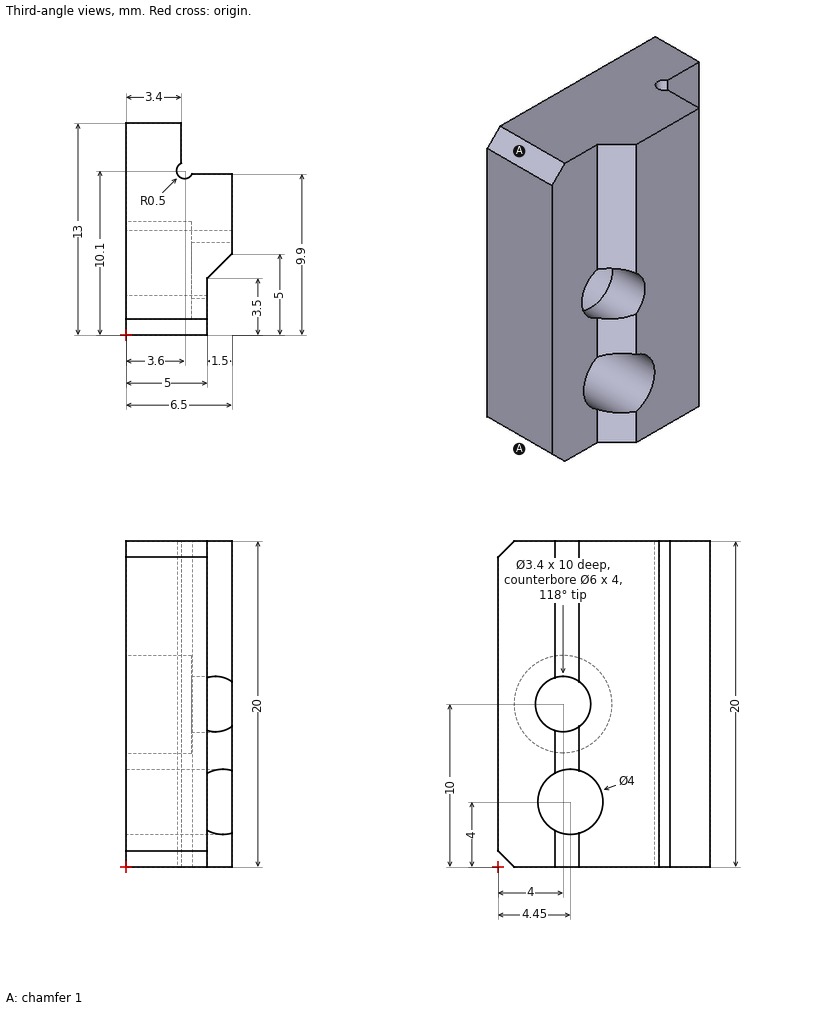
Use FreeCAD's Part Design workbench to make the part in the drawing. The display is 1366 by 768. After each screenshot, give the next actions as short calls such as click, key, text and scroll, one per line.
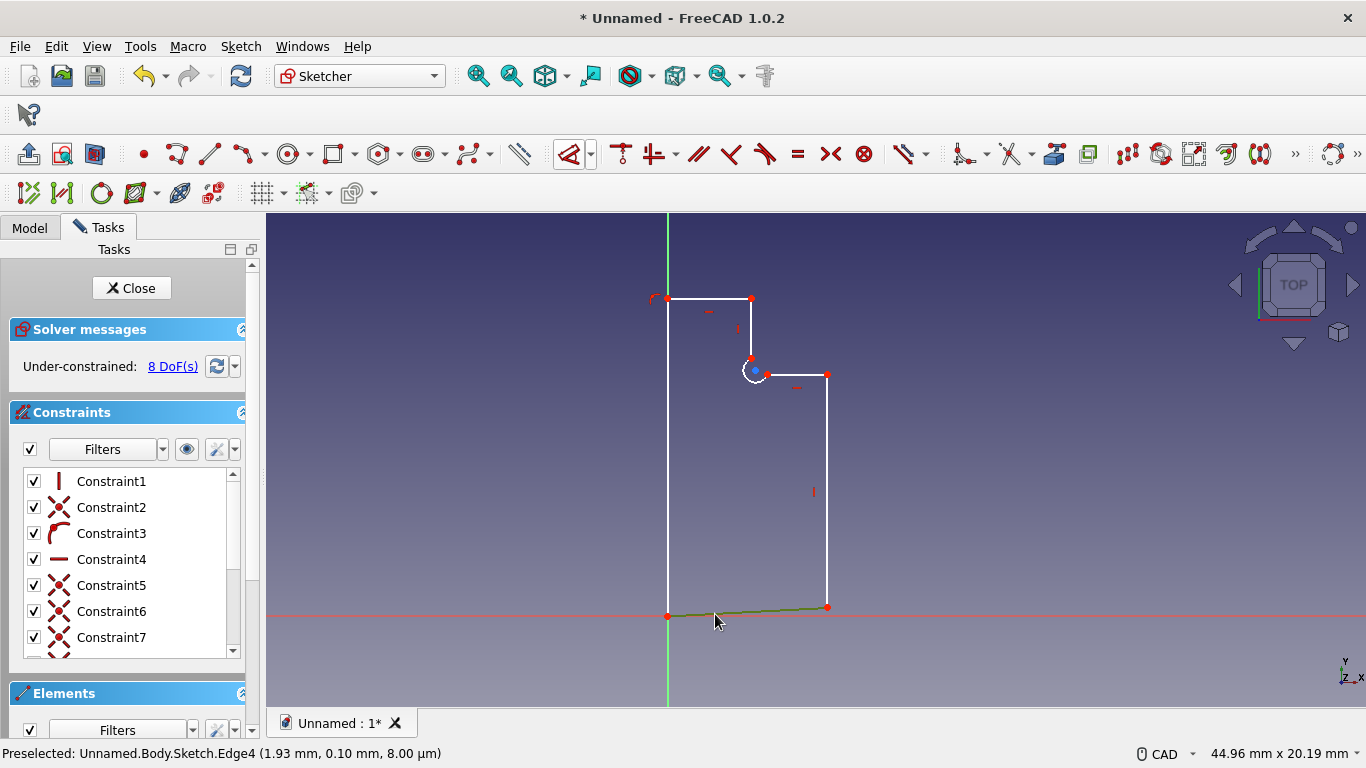
key(h)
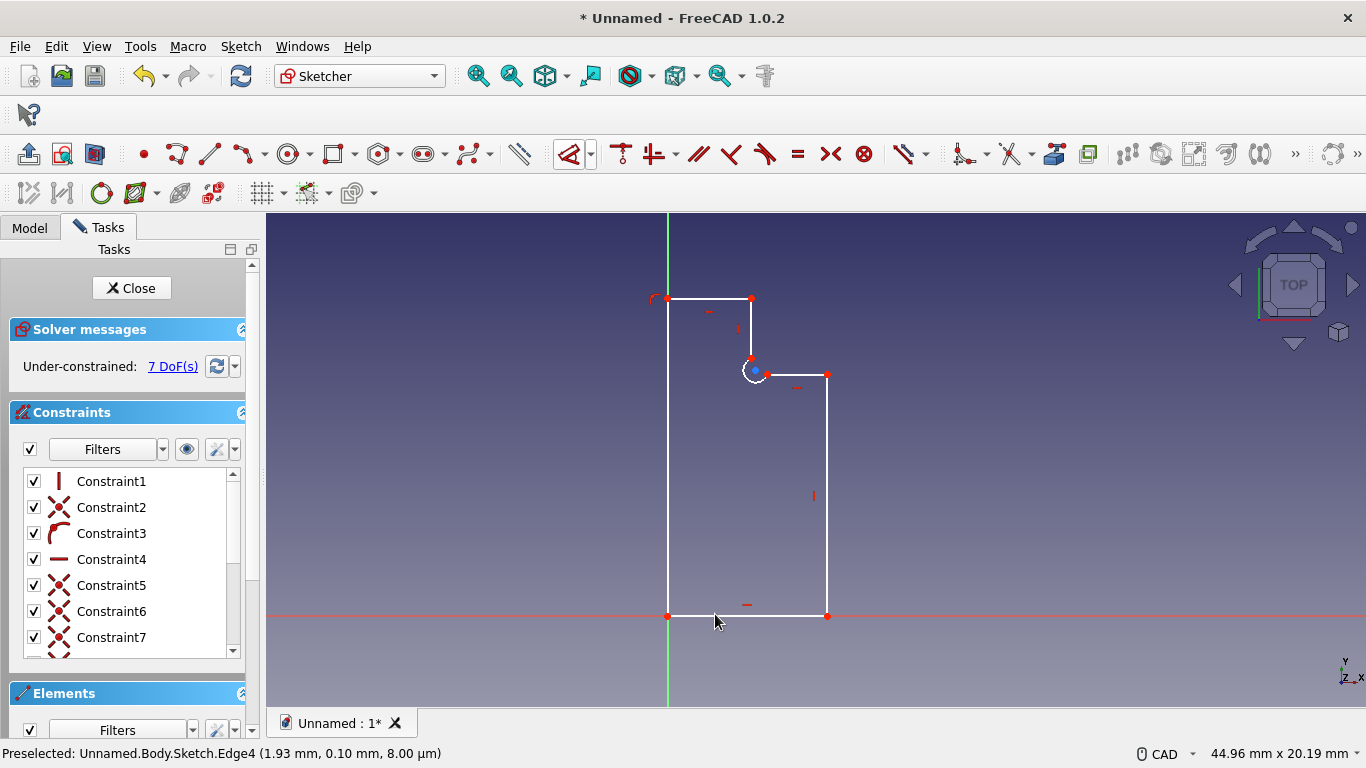
click(568, 154)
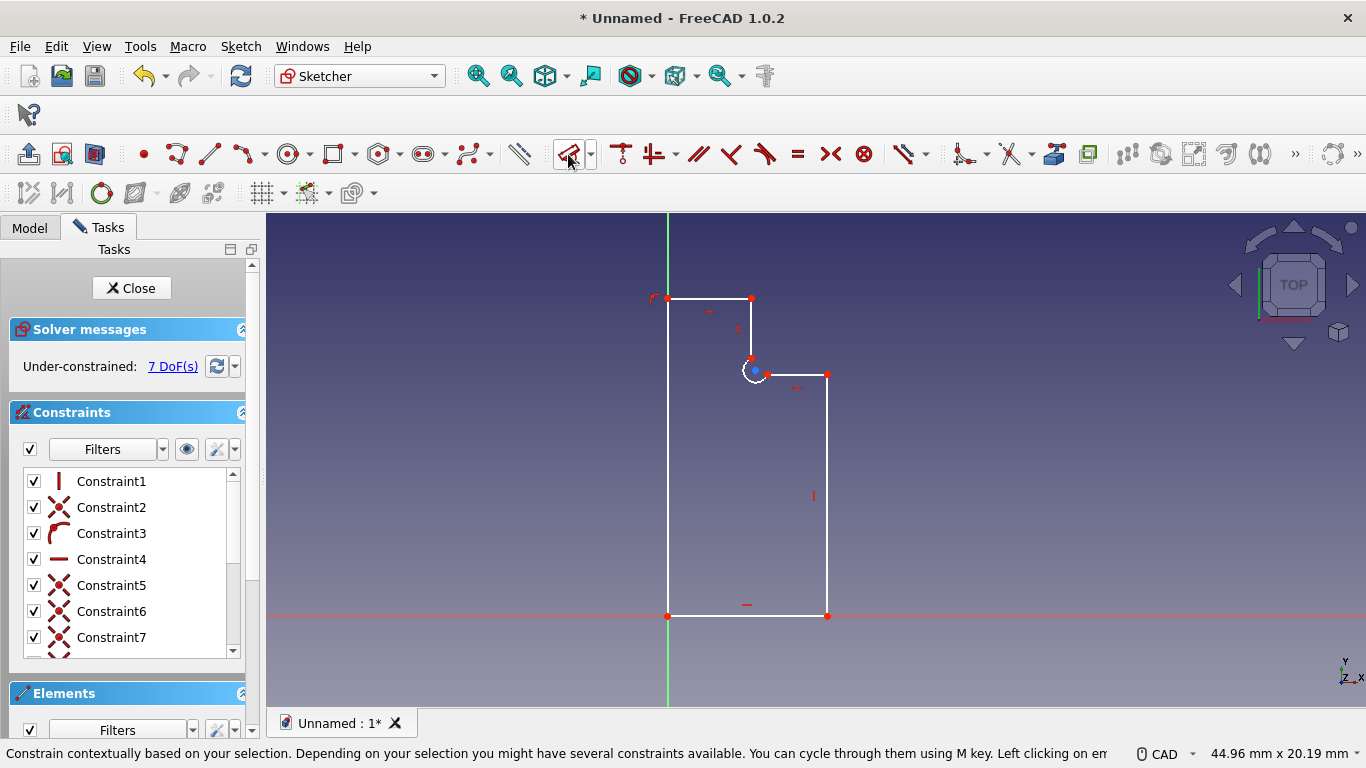
scroll(743, 370, up, 6)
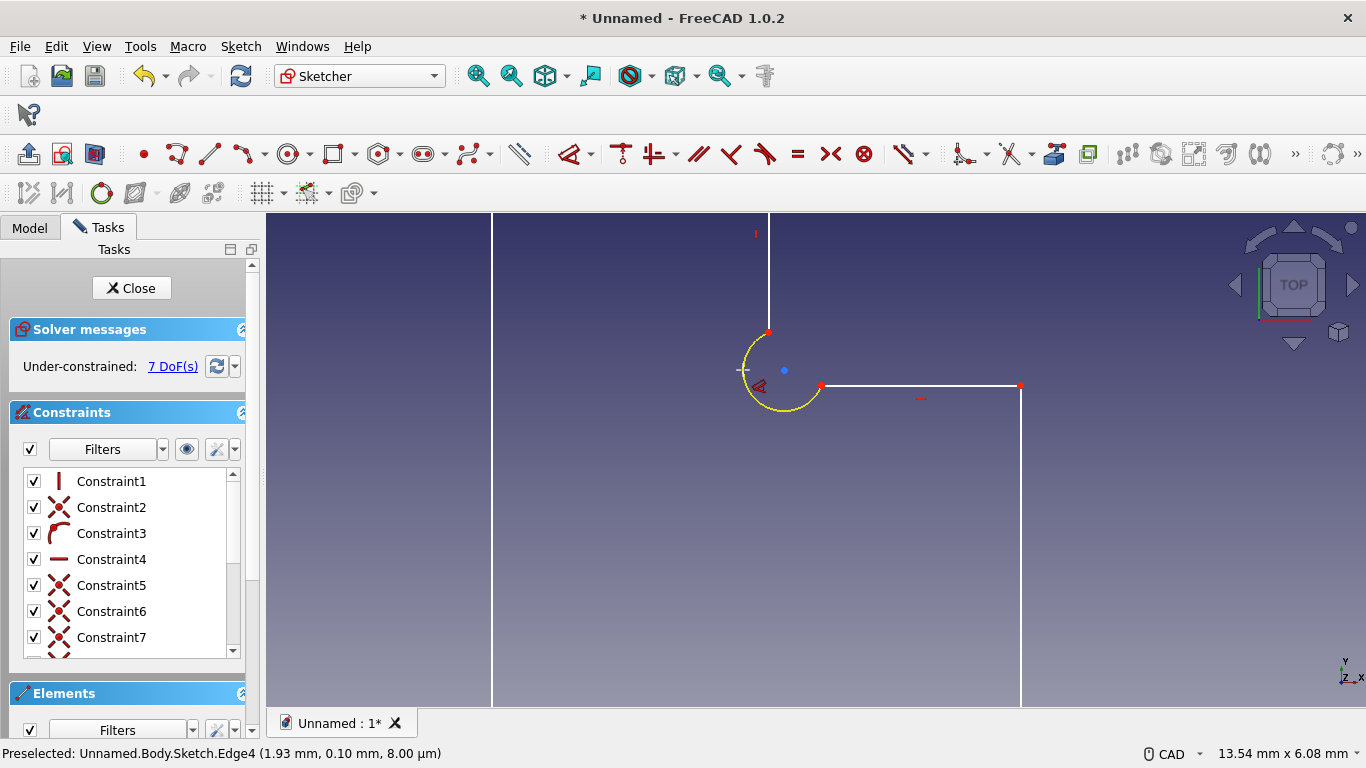
click(743, 370)
click(711, 370)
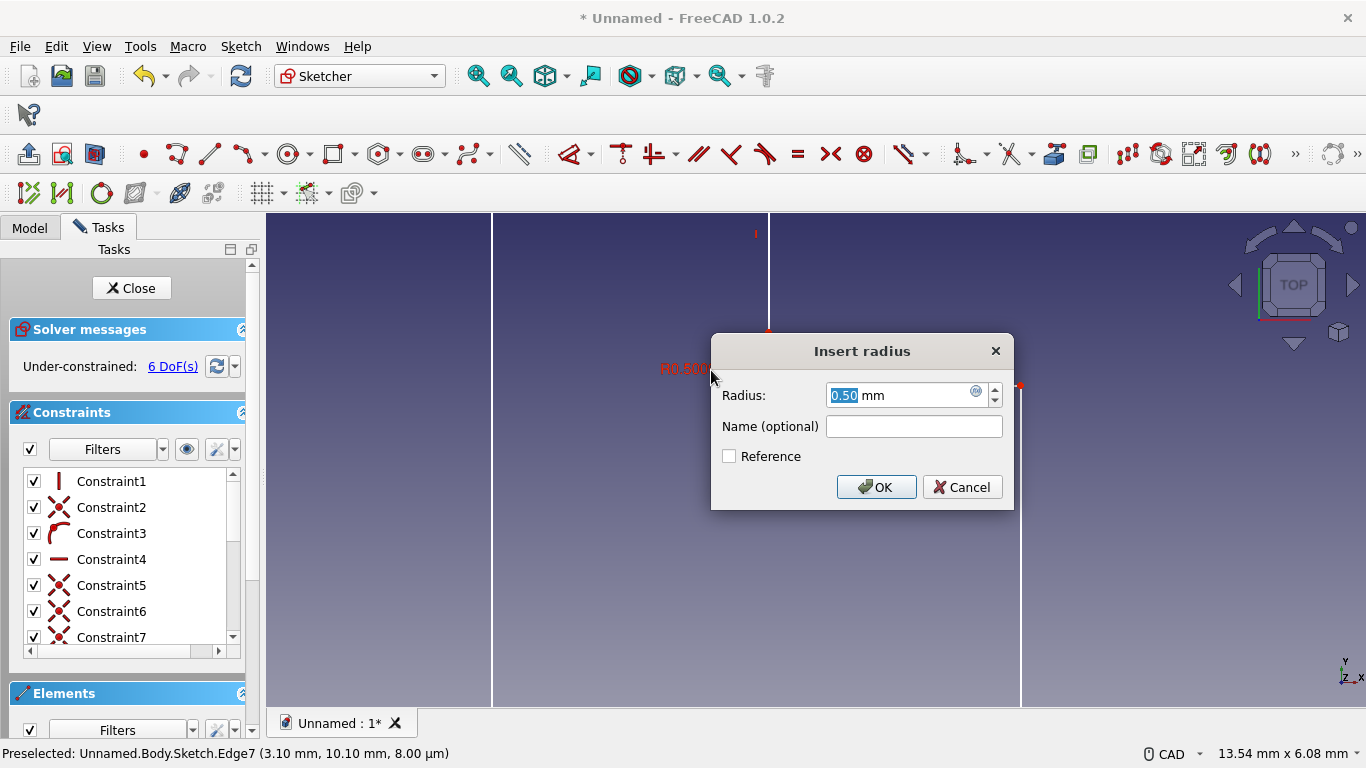
text(0.5)
key(Return)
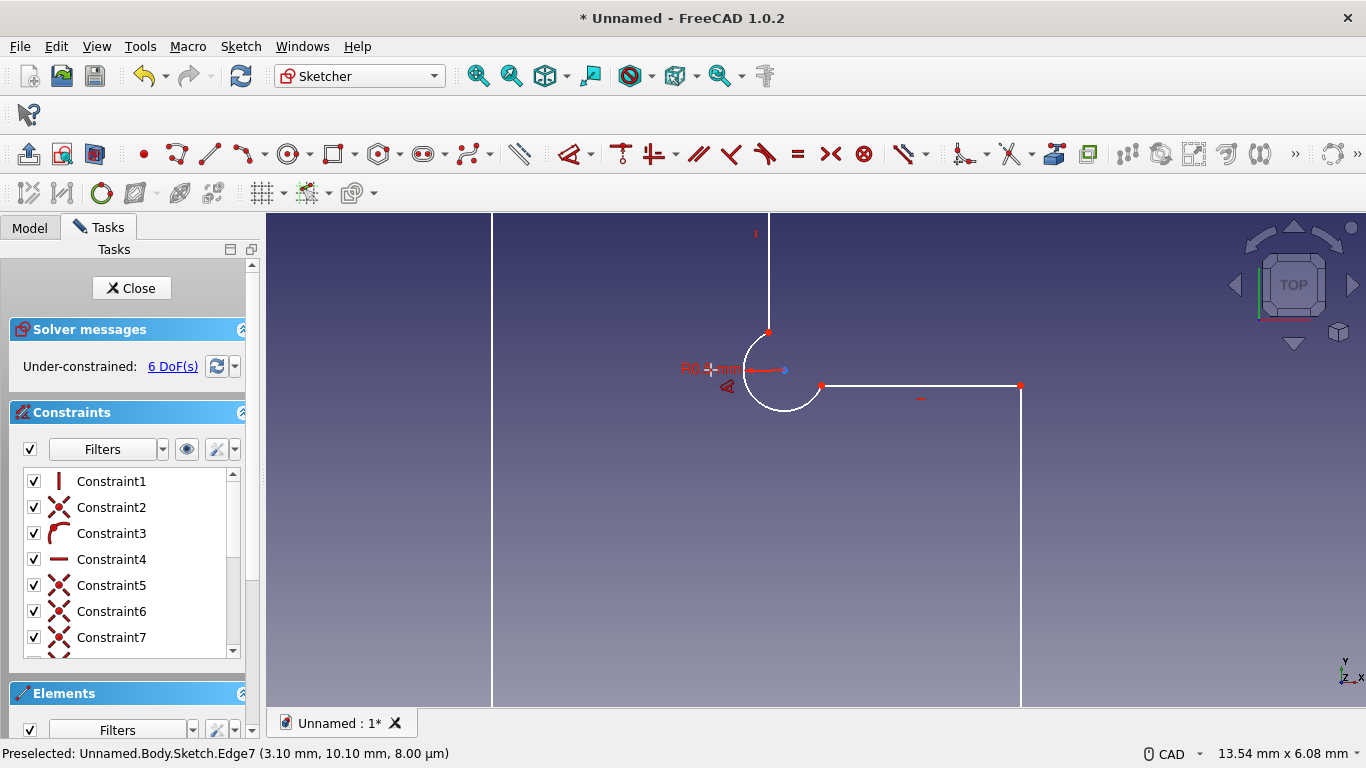
click(492, 450)
click(458, 460)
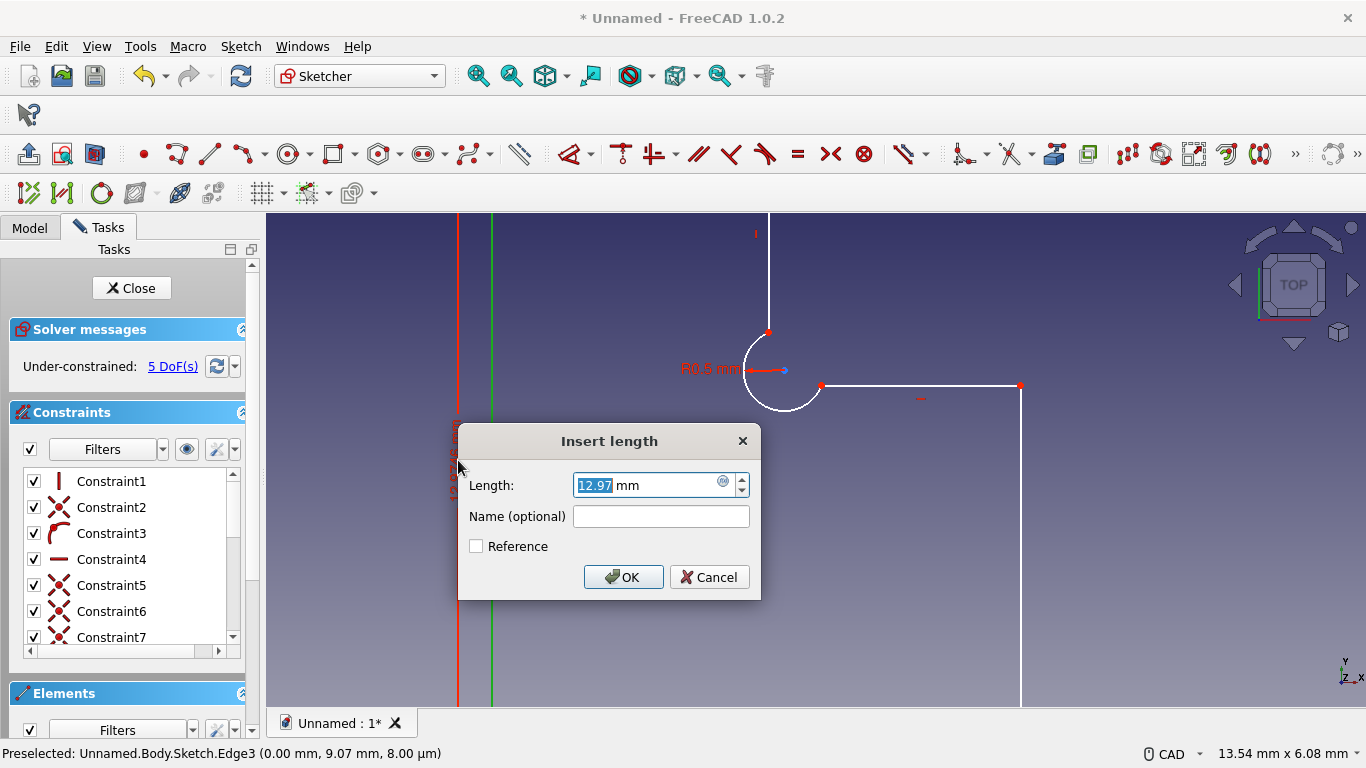
text(13)
key(Return)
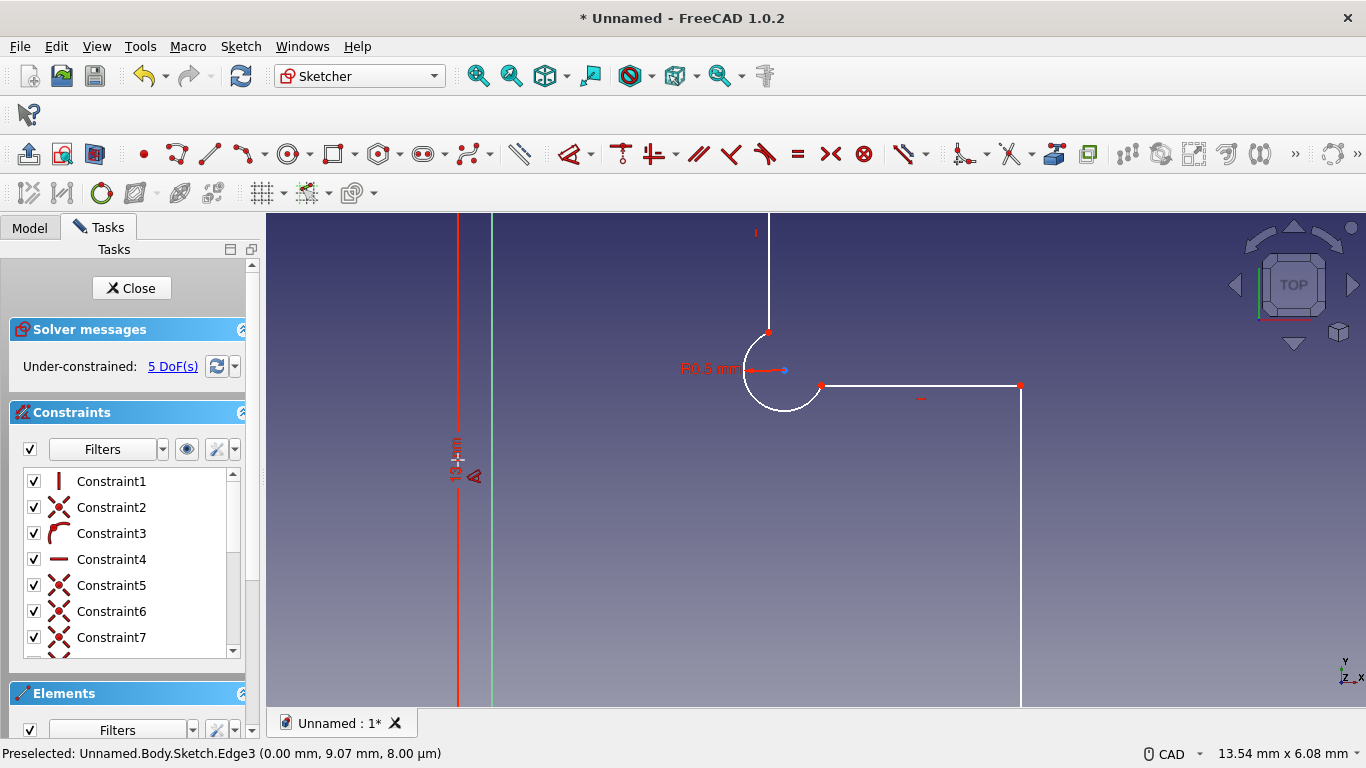
scroll(744, 374, down, 6)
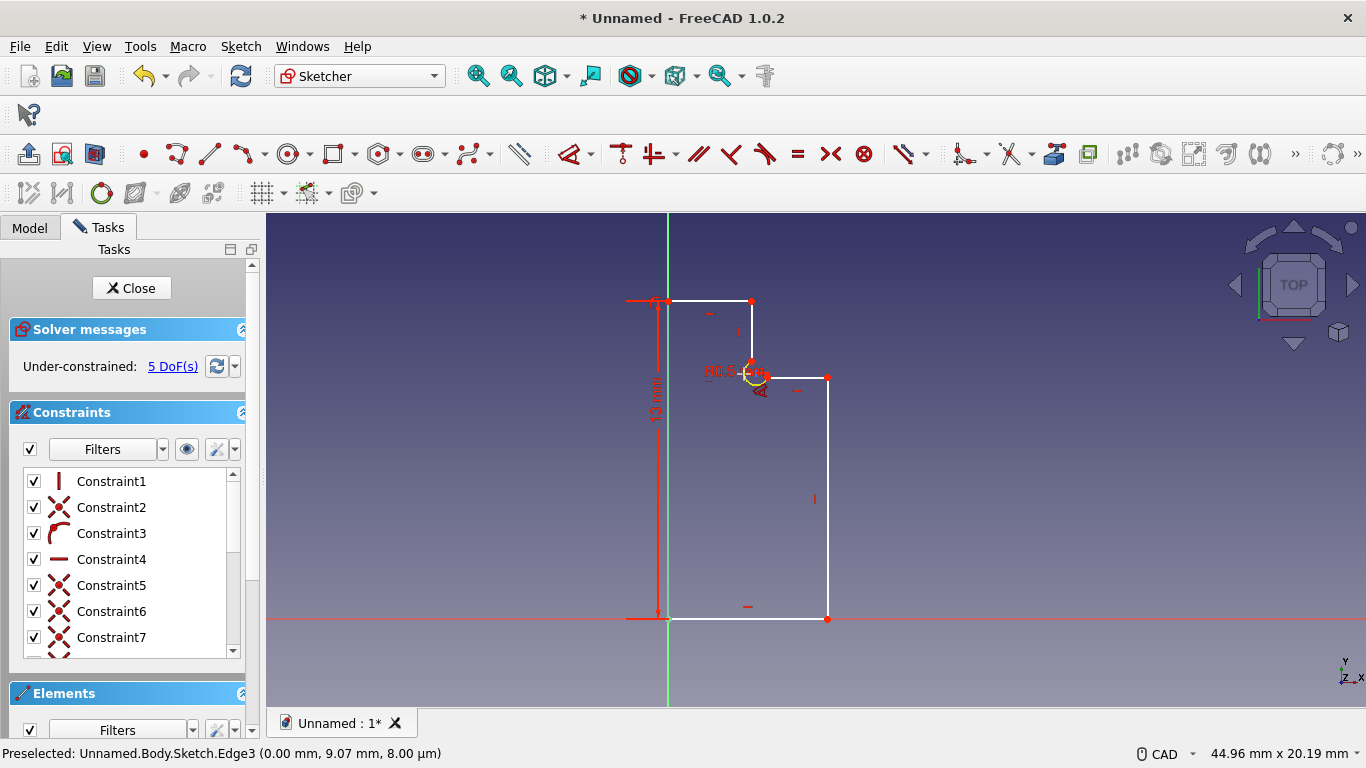
click(727, 301)
click(710, 267)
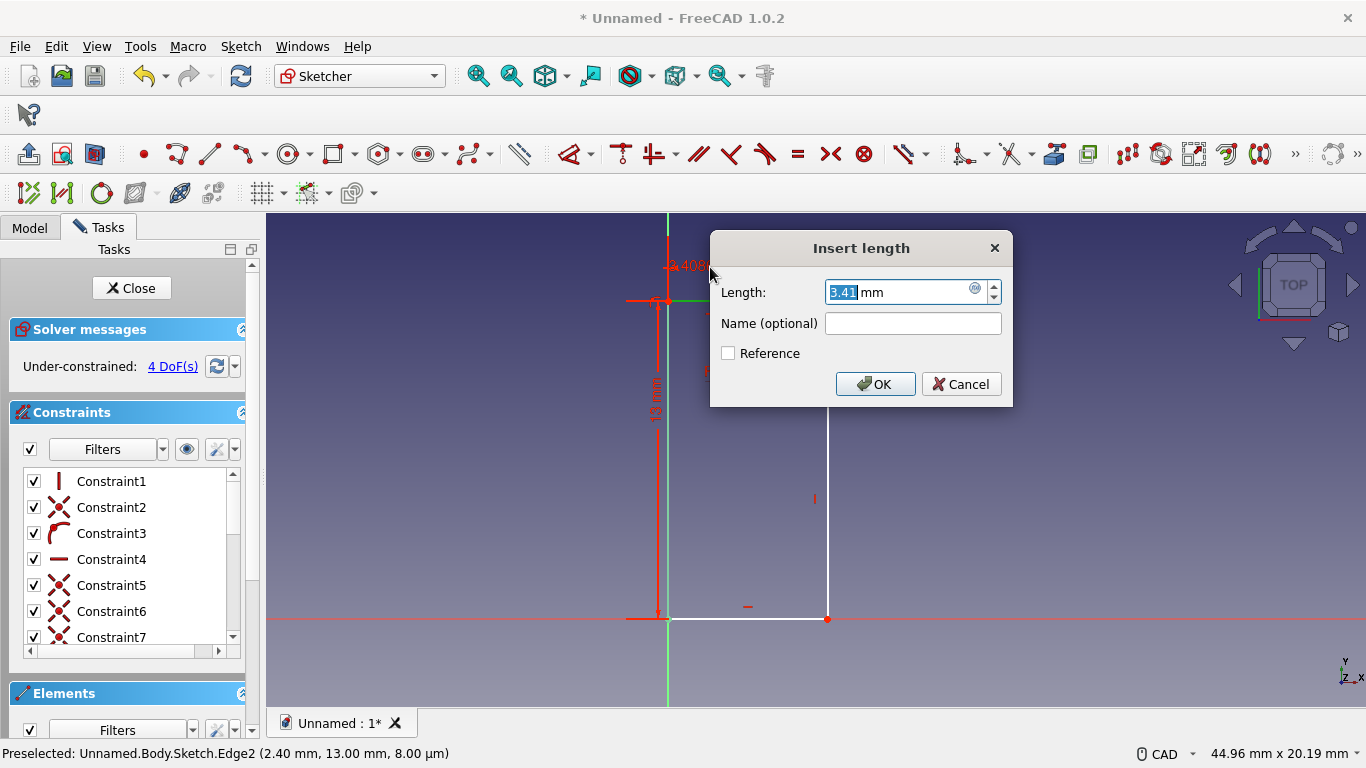
text(3.4)
key(Return)